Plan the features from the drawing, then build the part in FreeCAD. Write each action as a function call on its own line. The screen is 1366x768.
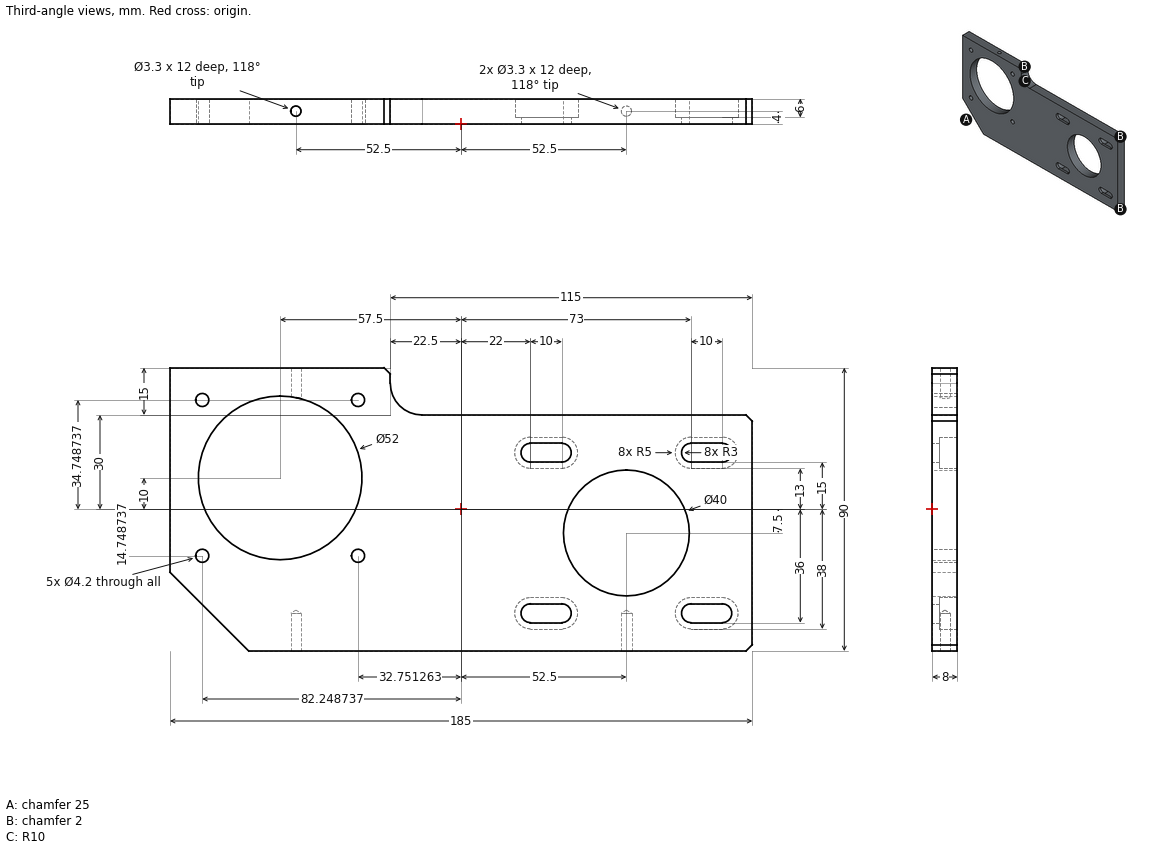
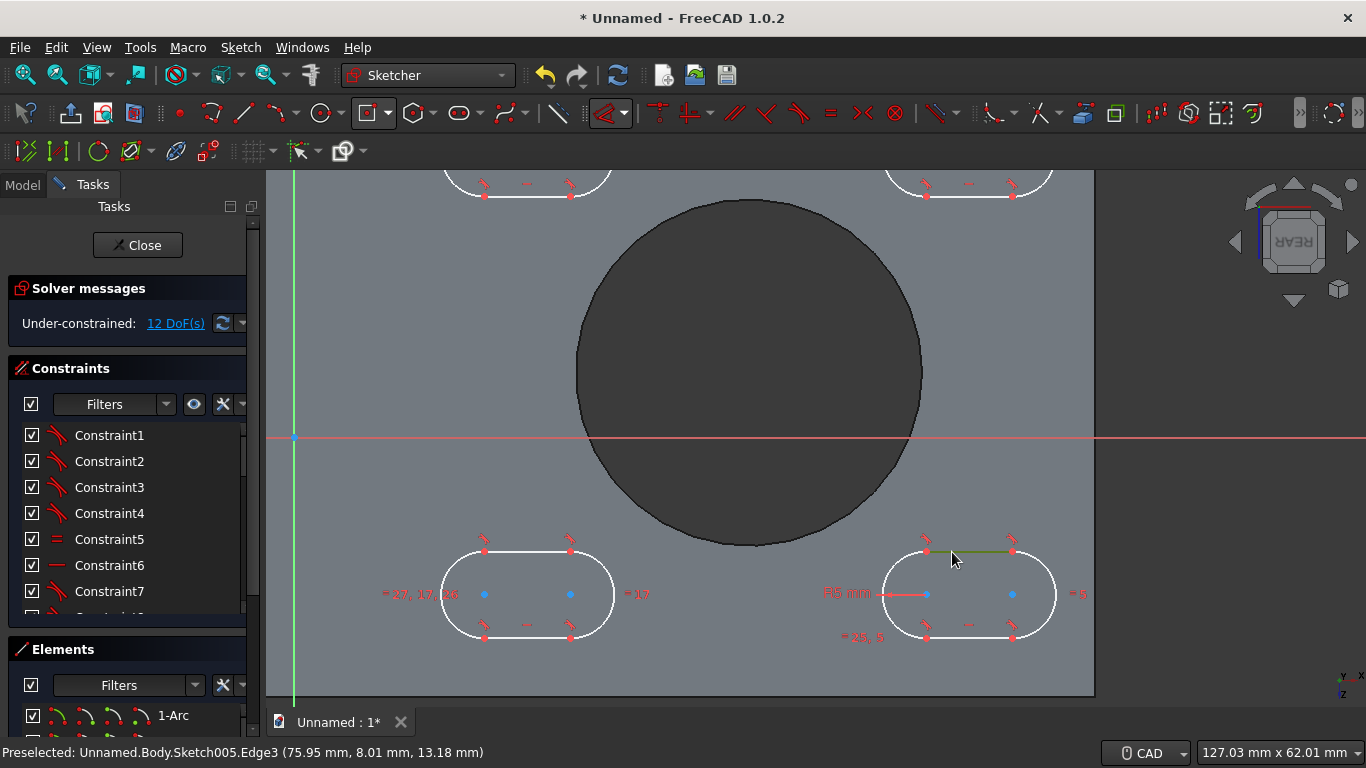
click(626, 114)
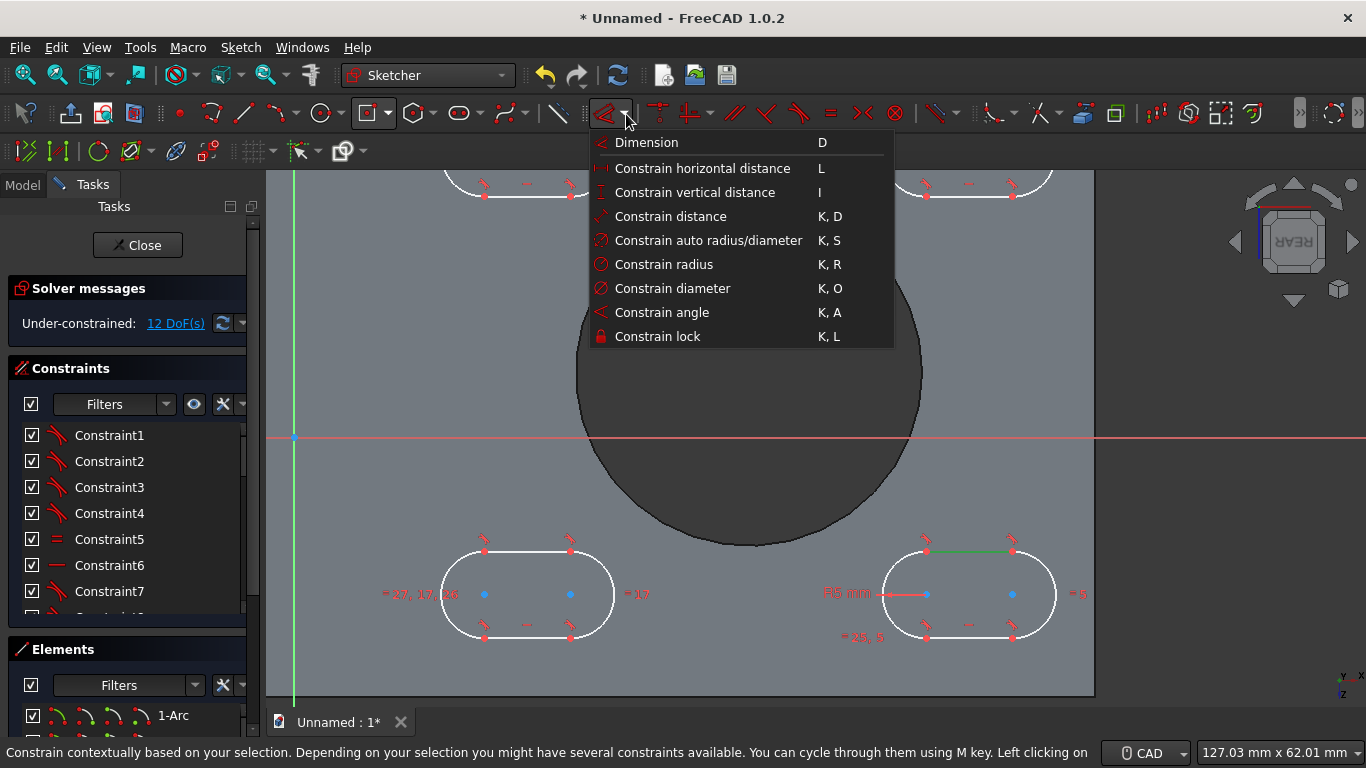
click(742, 168)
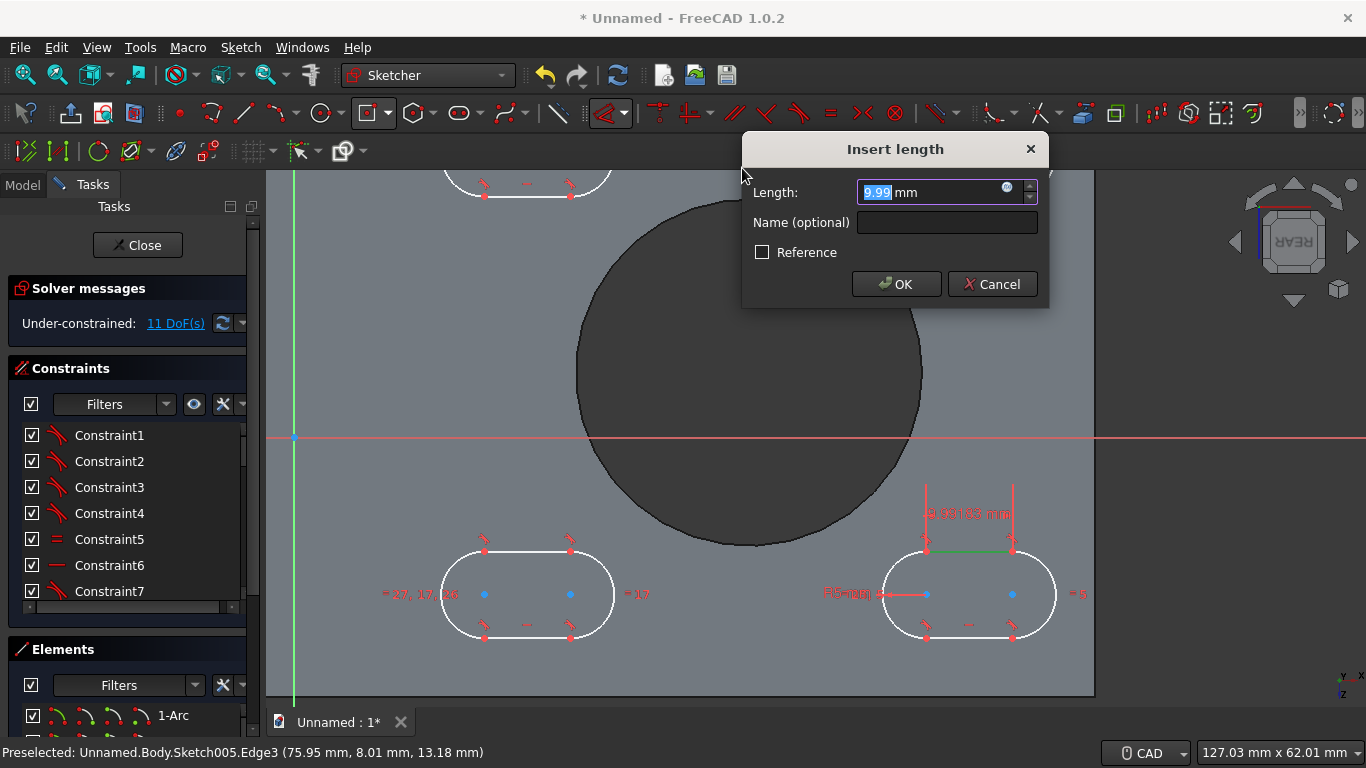
text(10)
key(Return)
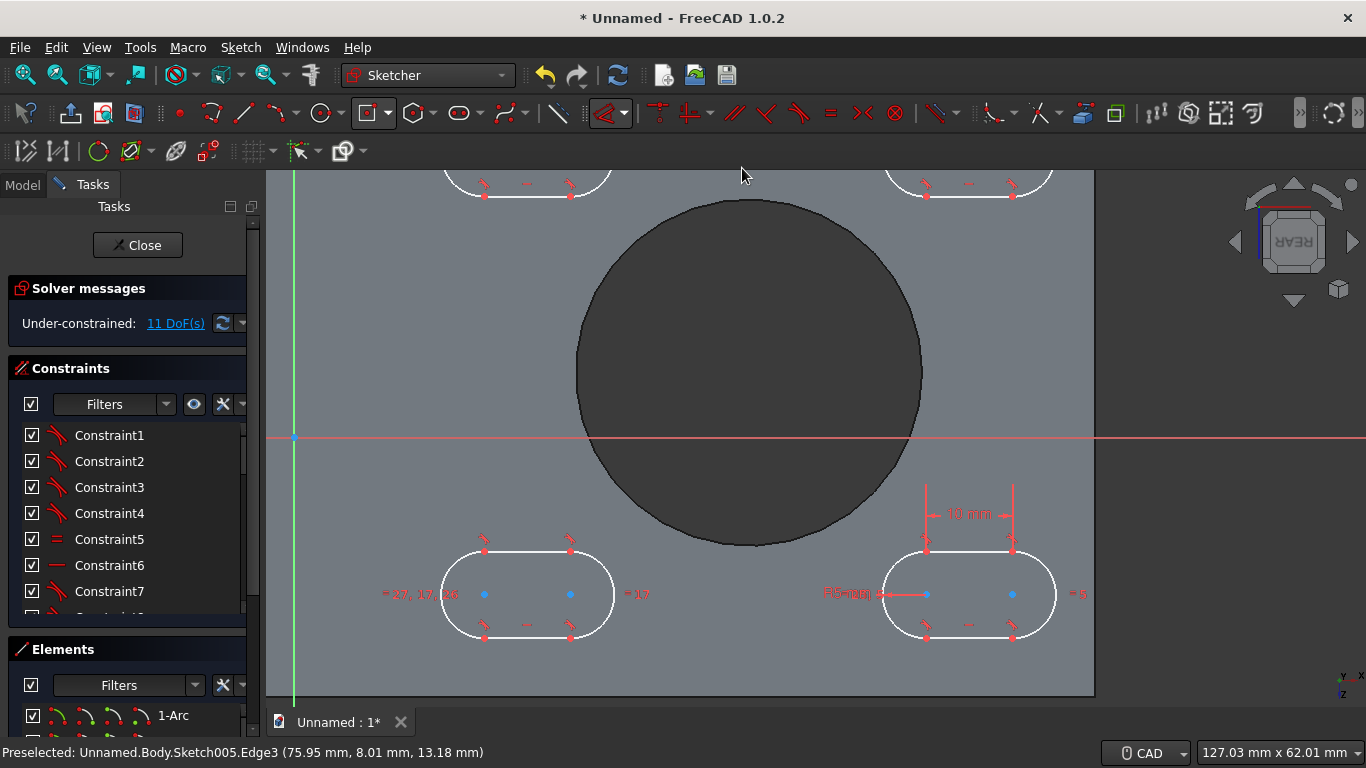
scroll(894, 572, down, 2)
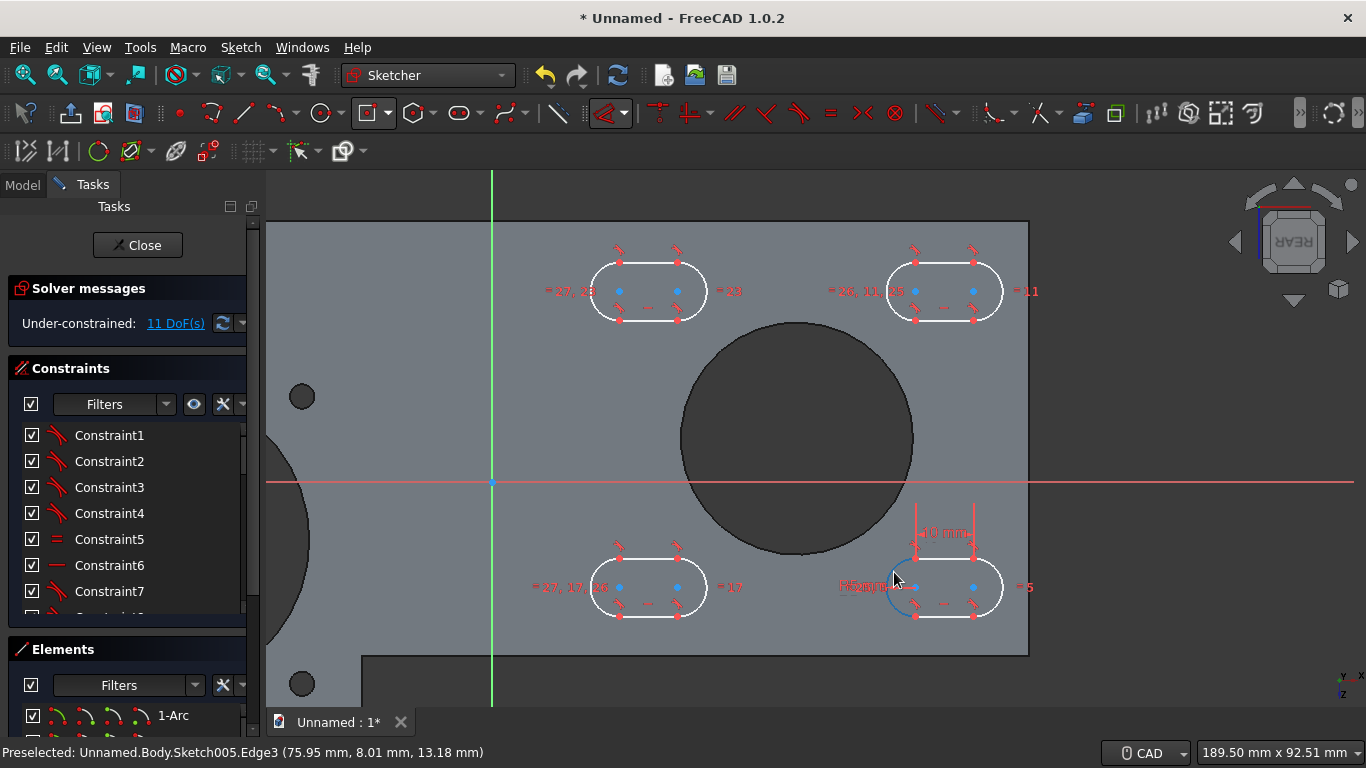
click(933, 263)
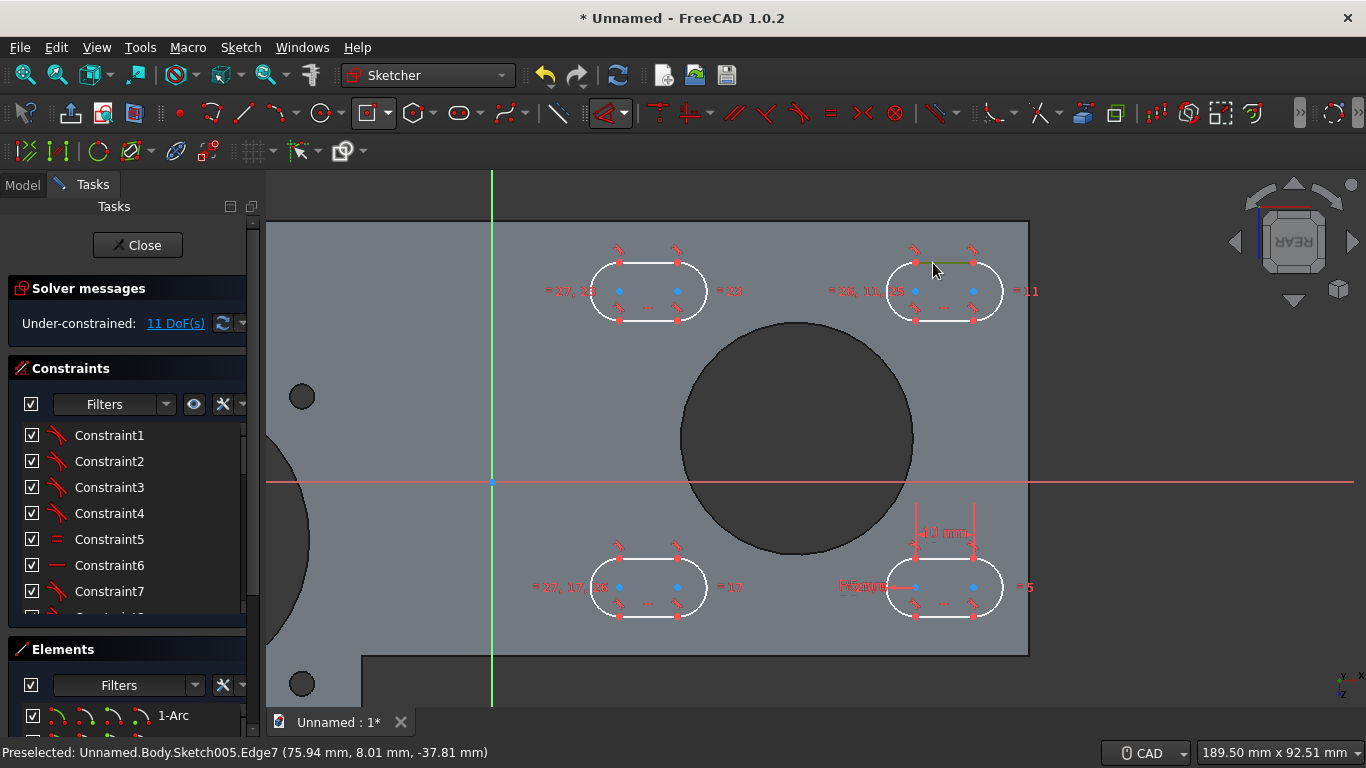
key(l)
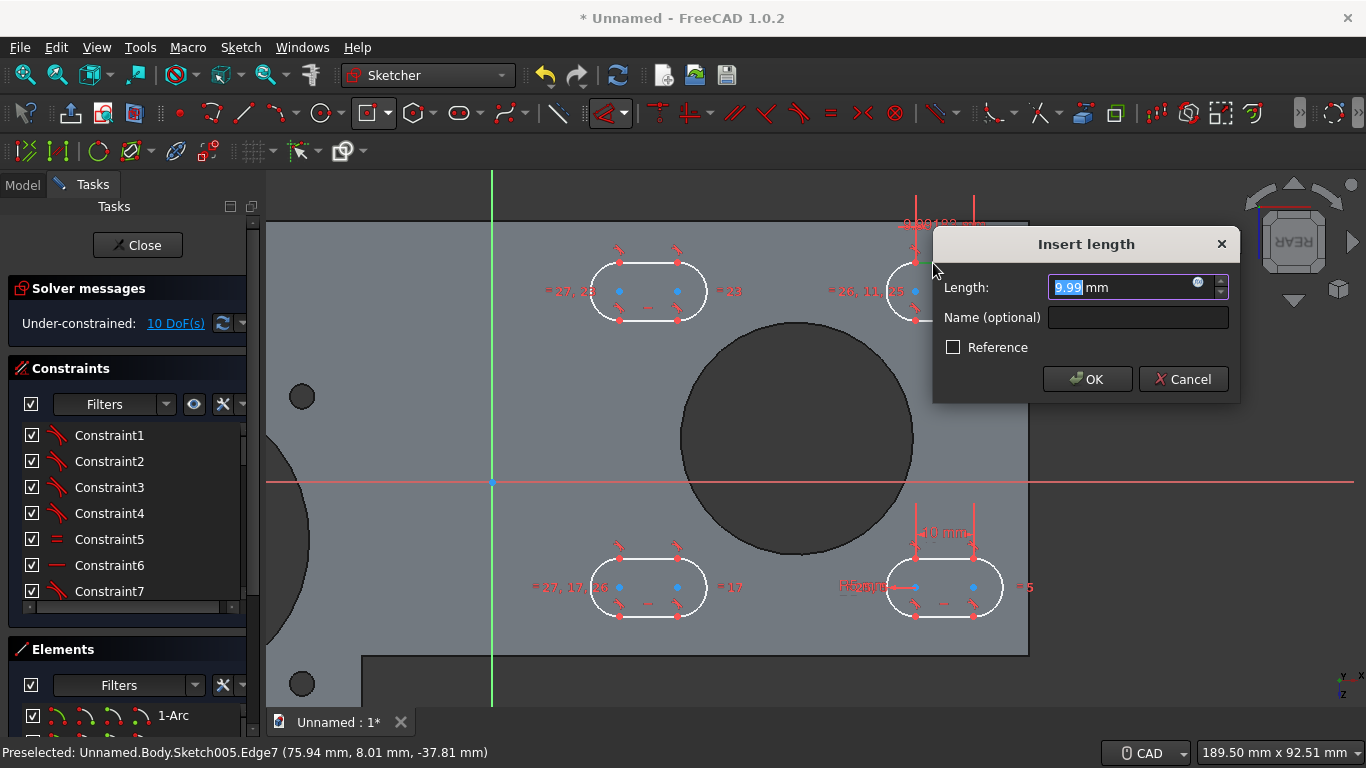
text(10)
key(Return)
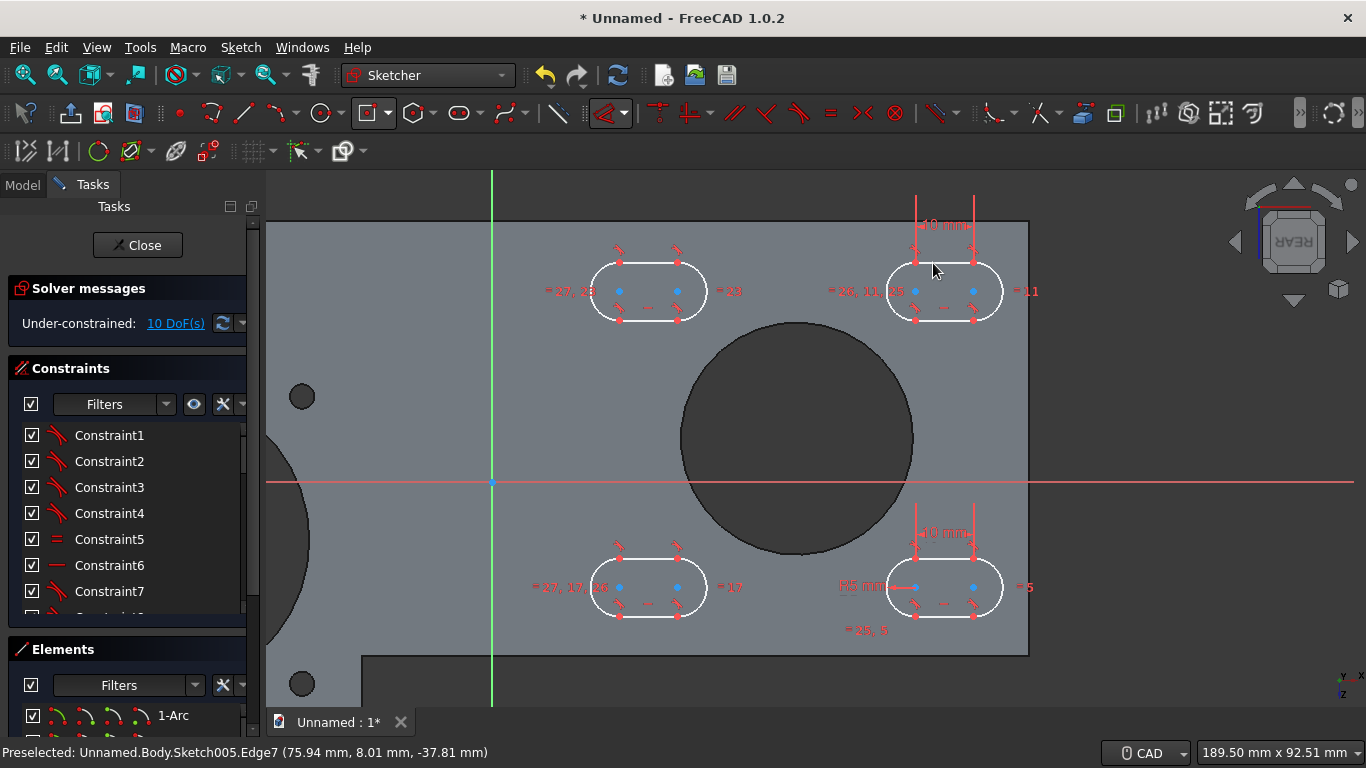
click(637, 559)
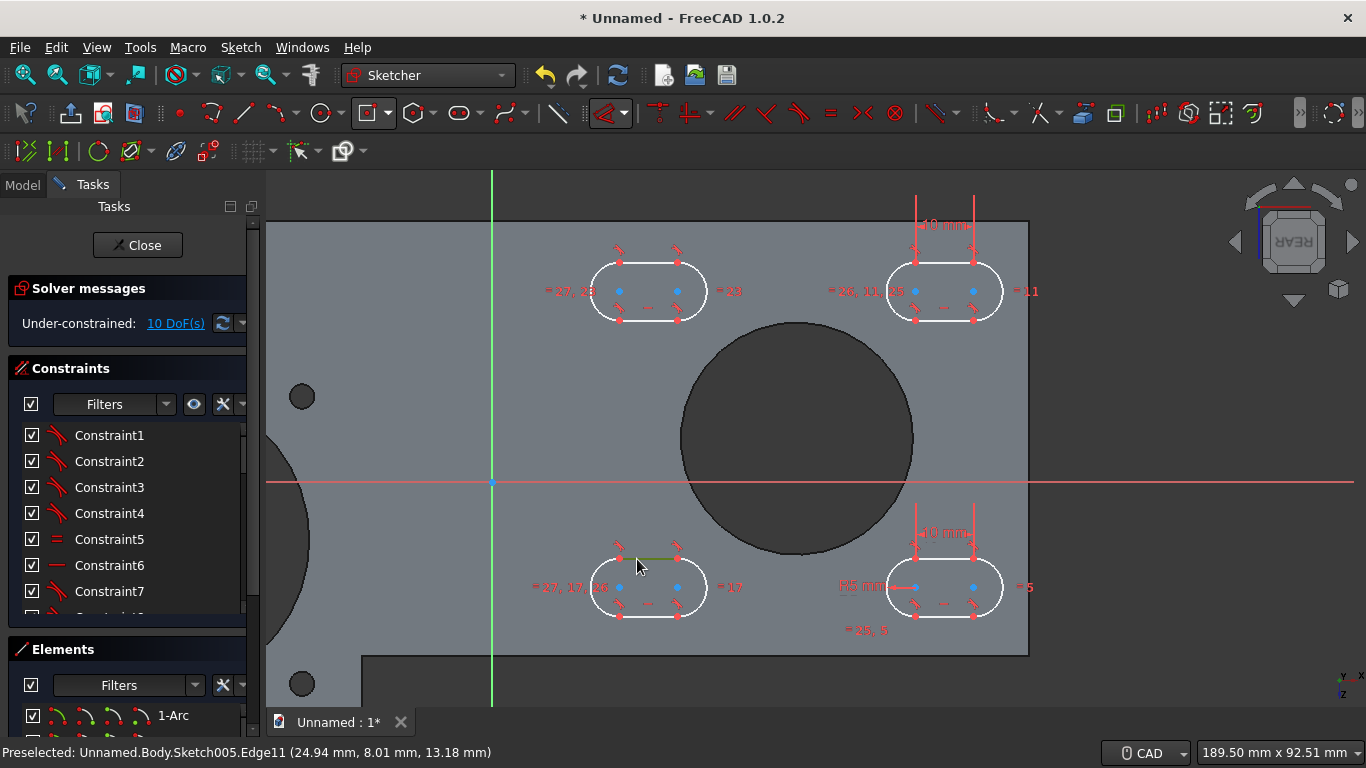
key(l)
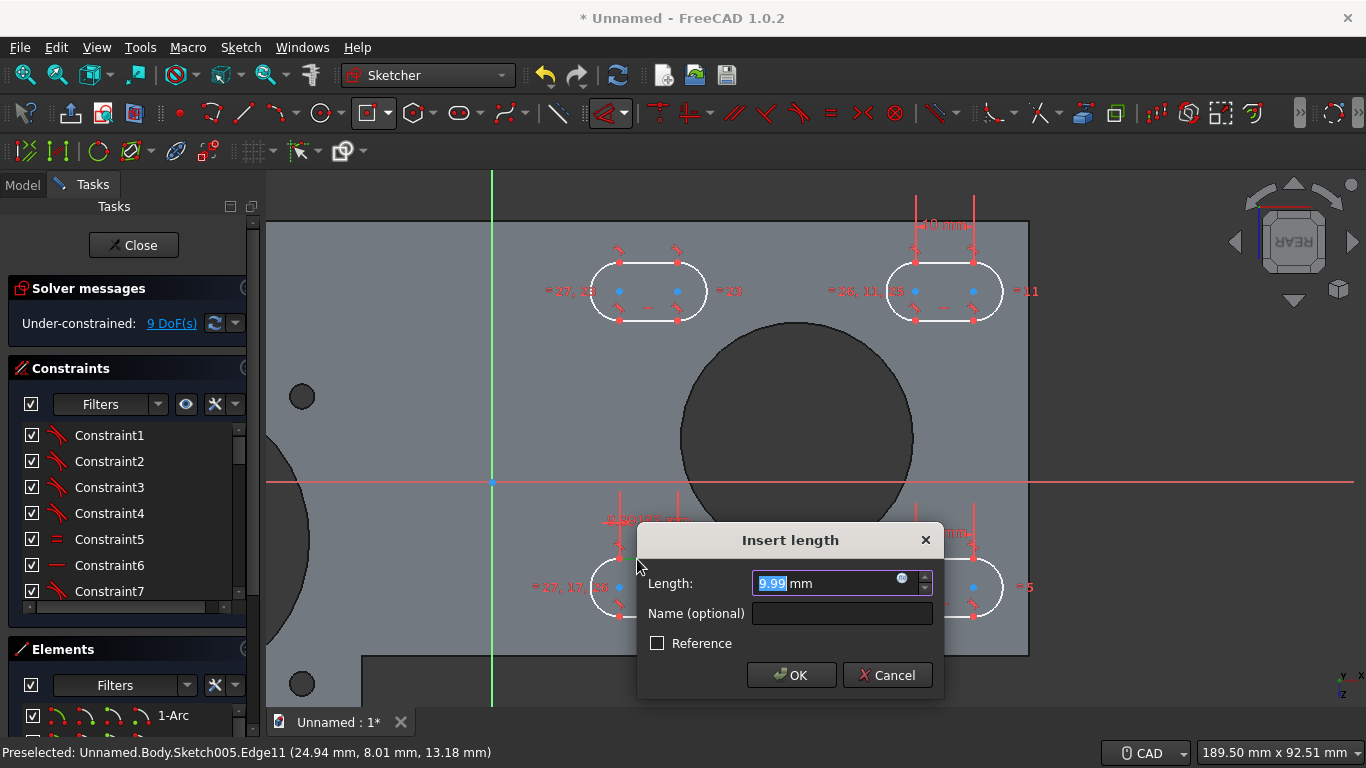
text(10)
key(Return)